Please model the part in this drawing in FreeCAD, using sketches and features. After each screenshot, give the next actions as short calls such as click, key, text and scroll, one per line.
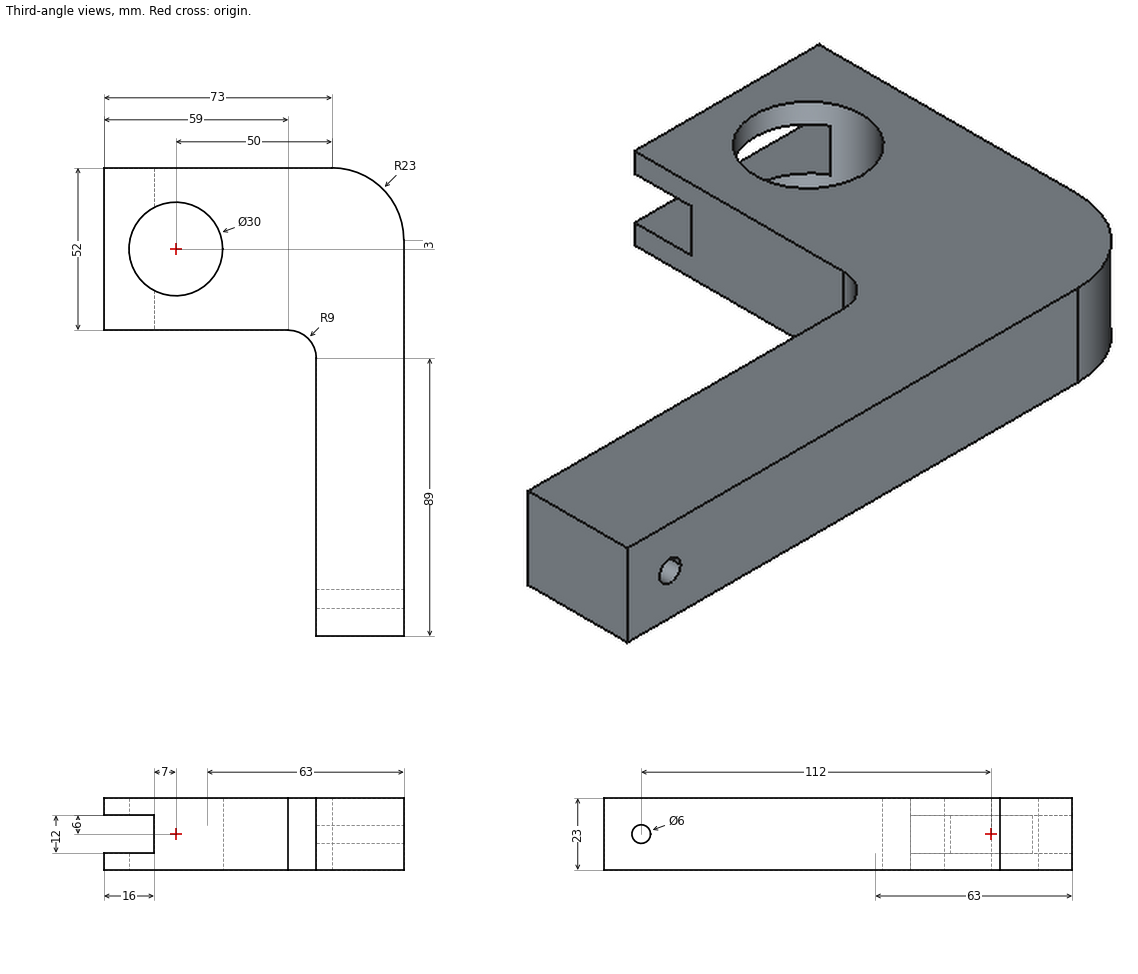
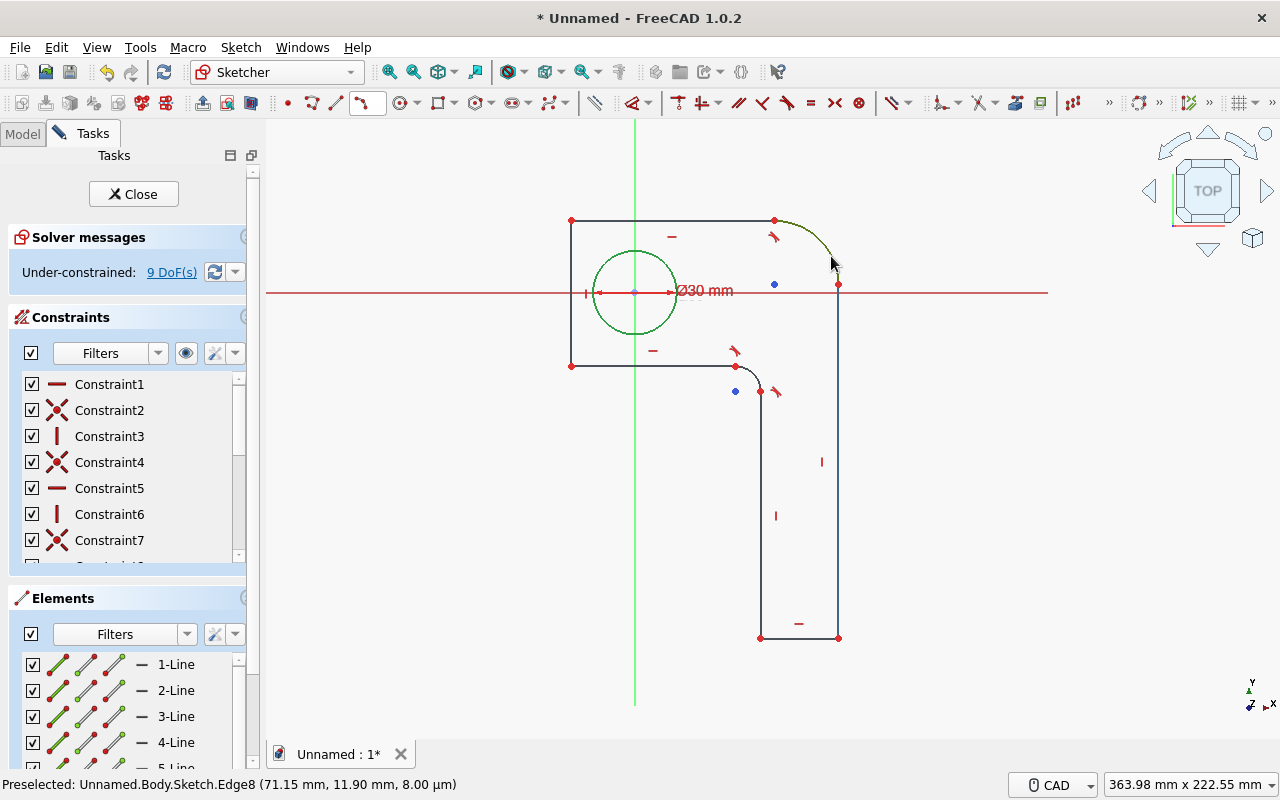
click(788, 104)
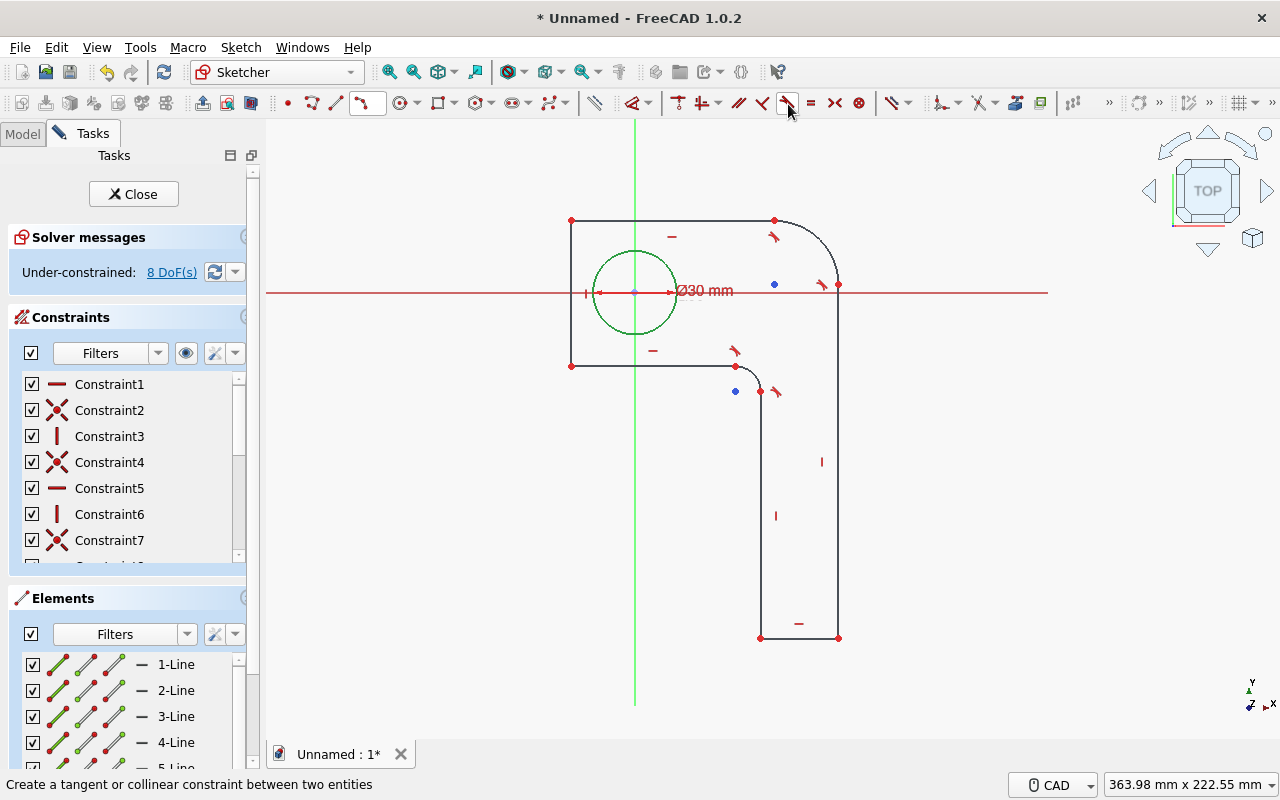
click(632, 104)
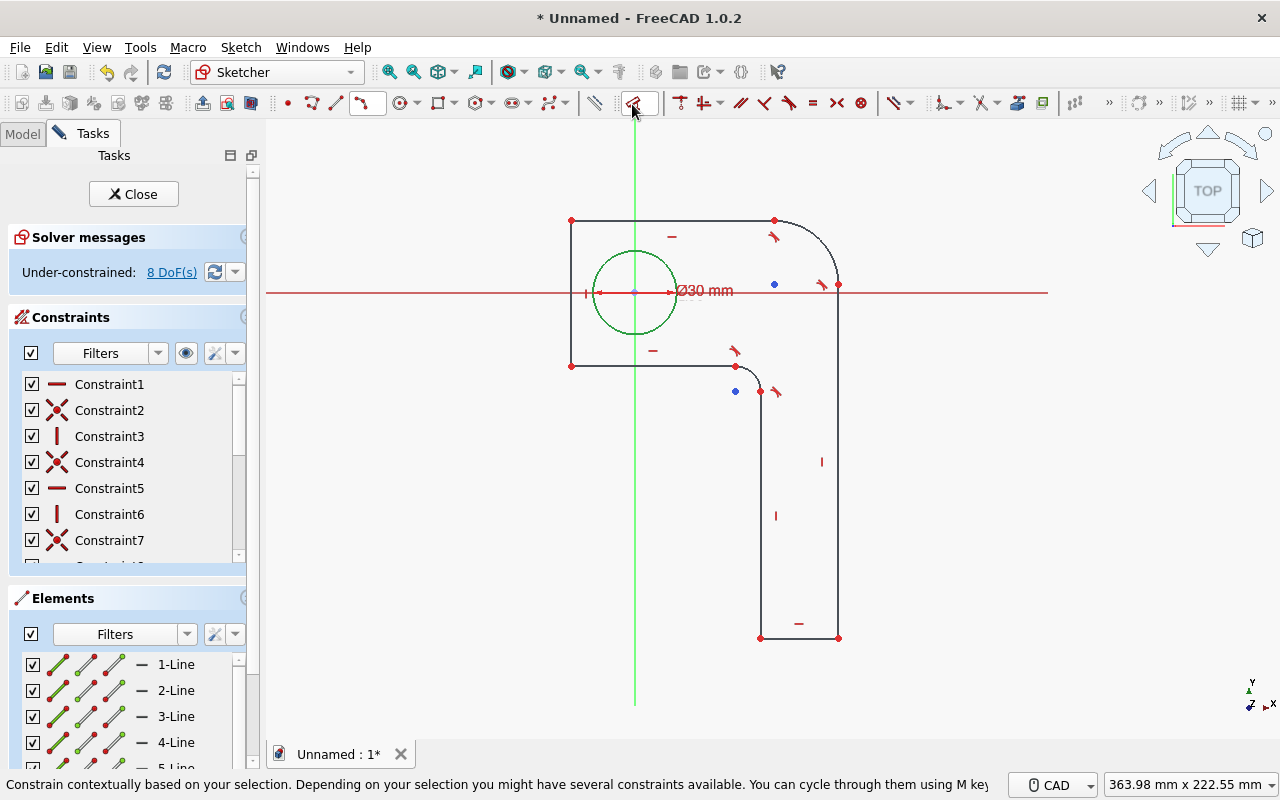
scroll(758, 380, up, 3)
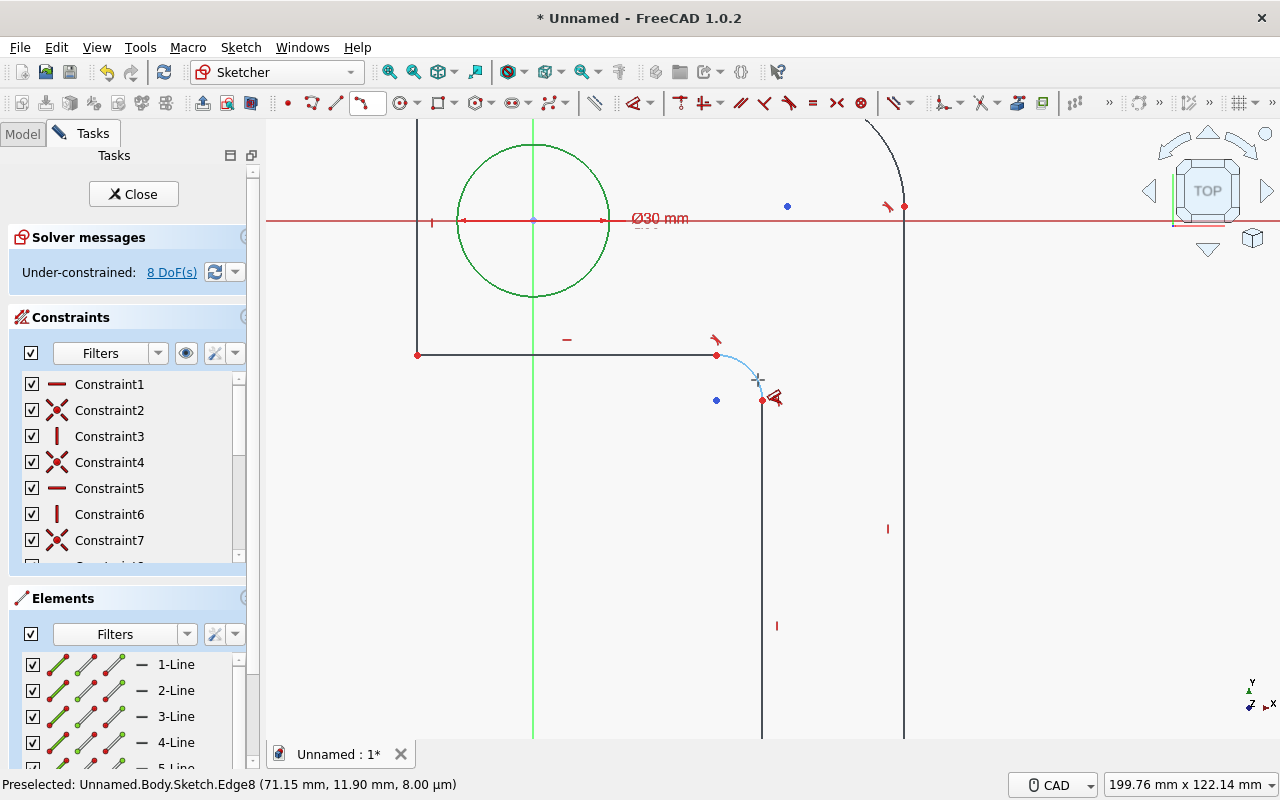
click(757, 380)
click(785, 365)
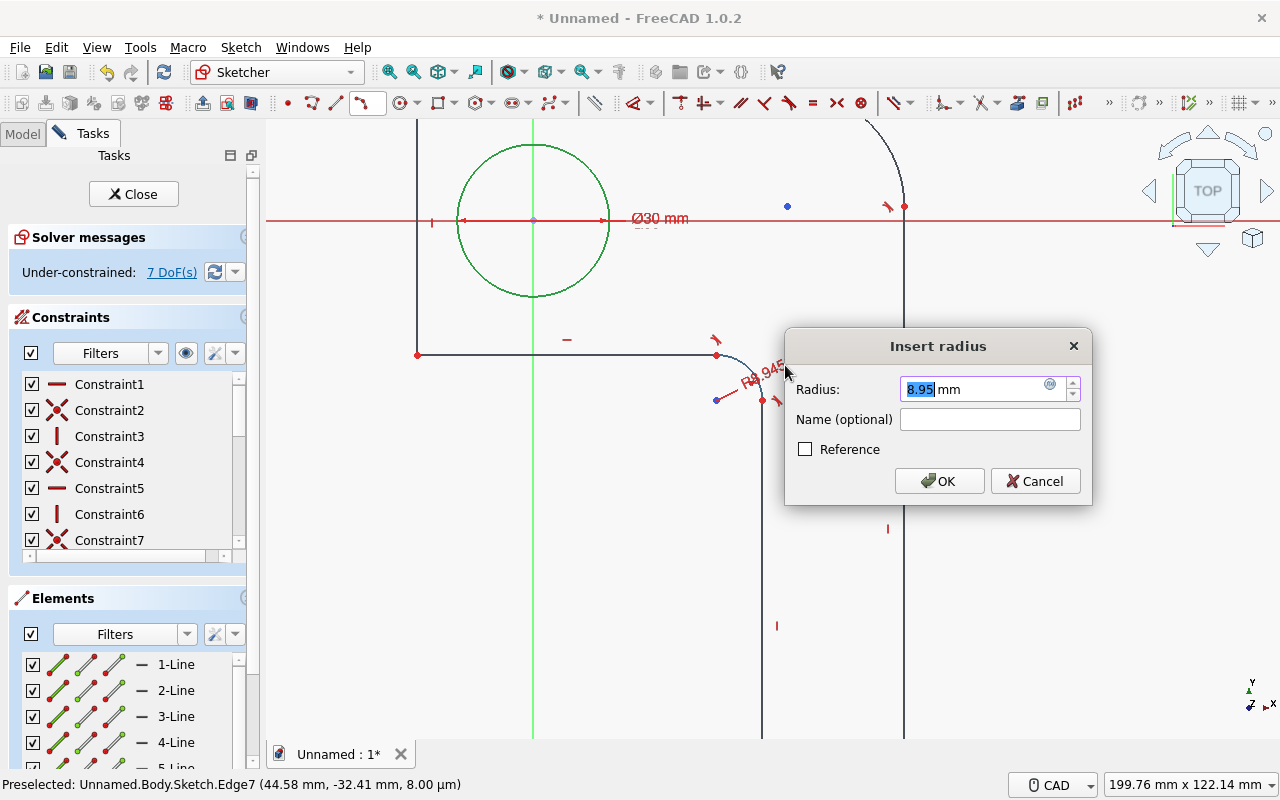
text(9)
key(Return)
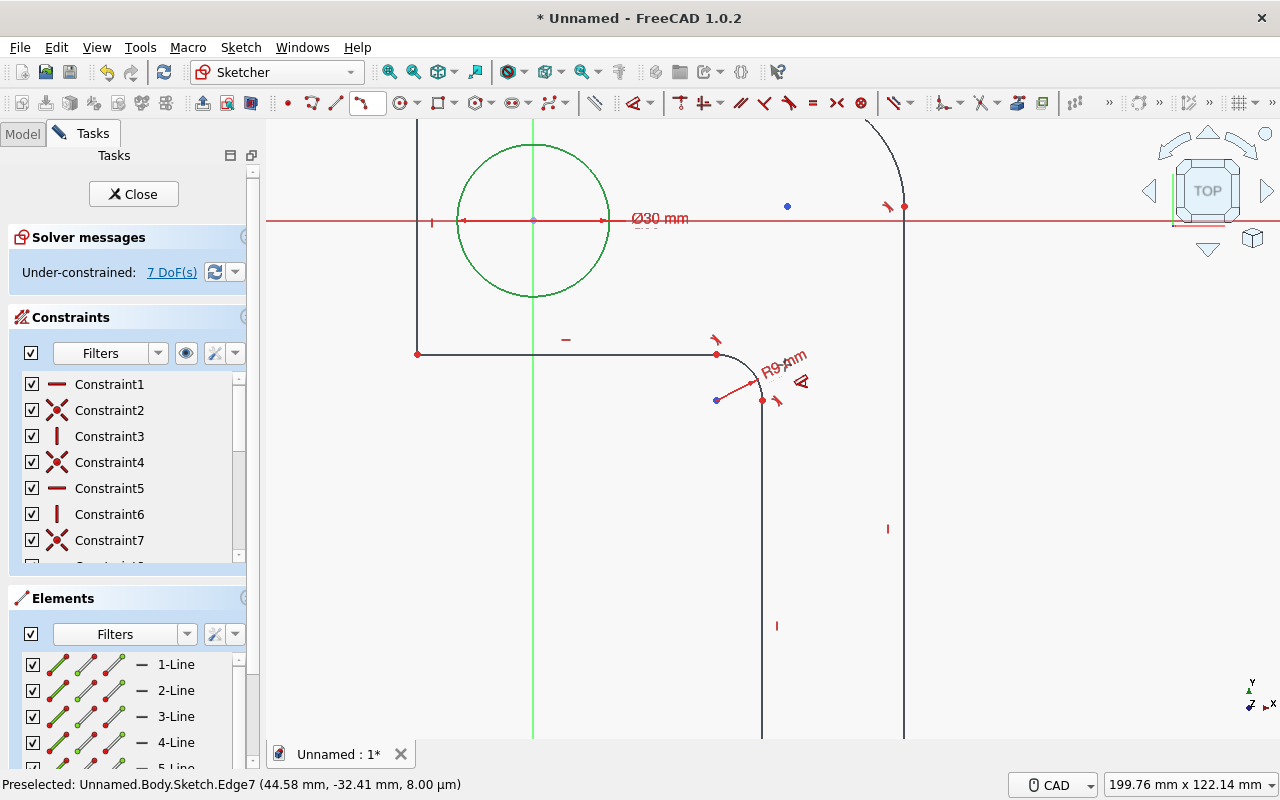
click(892, 153)
click(856, 339)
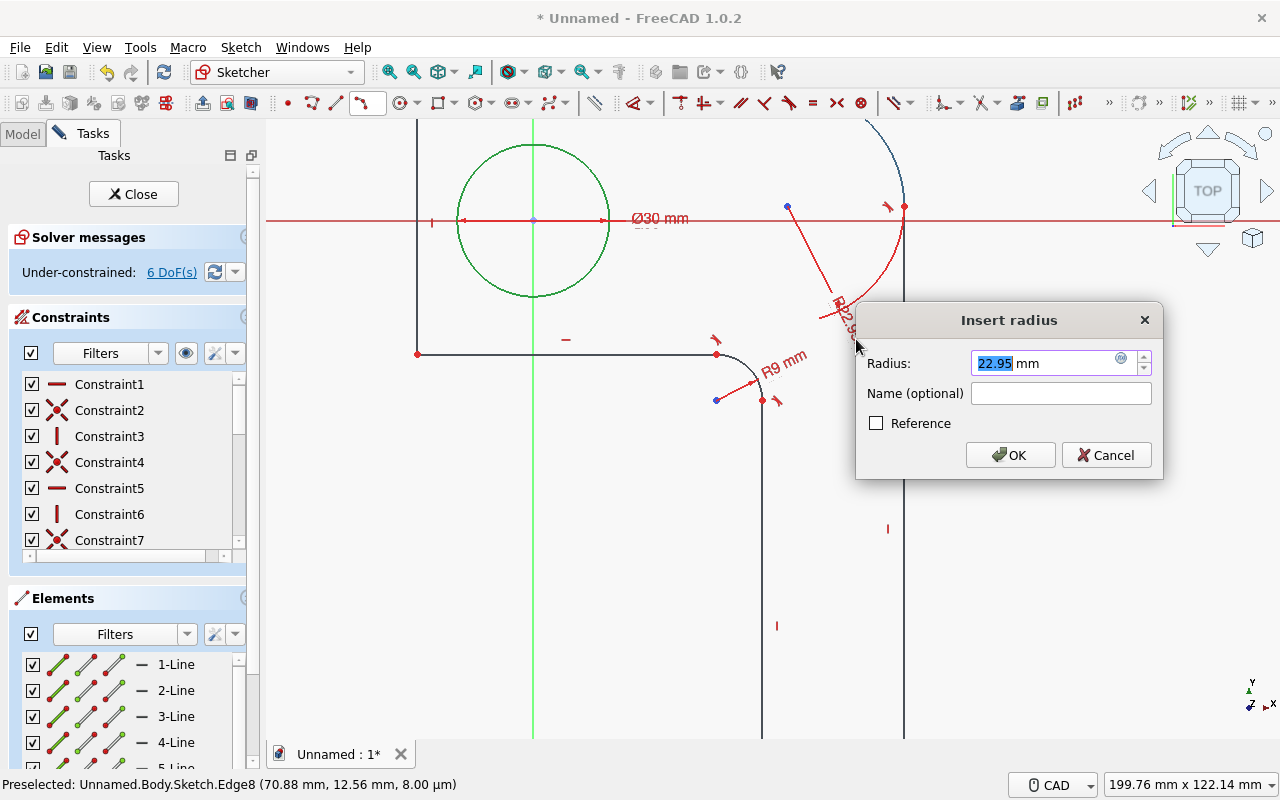
text(23)
key(Return)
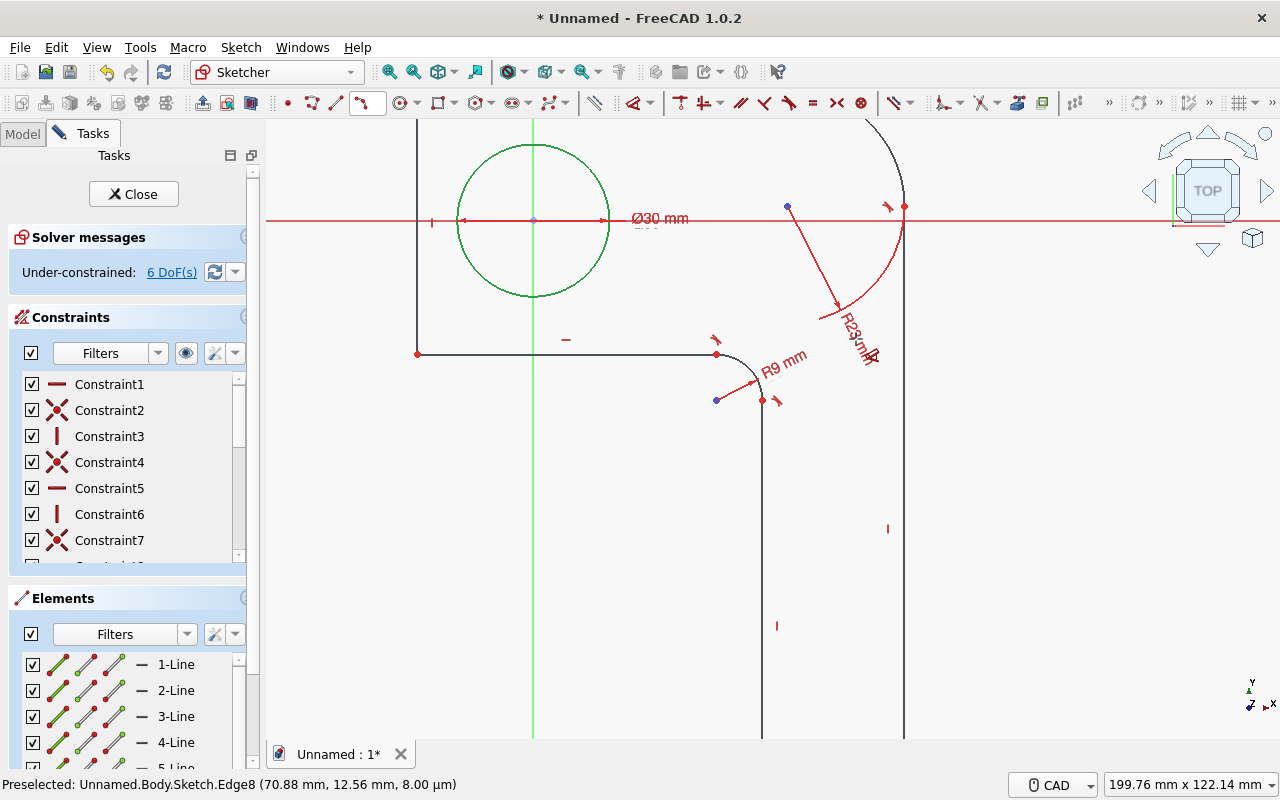
scroll(758, 380, down, 3)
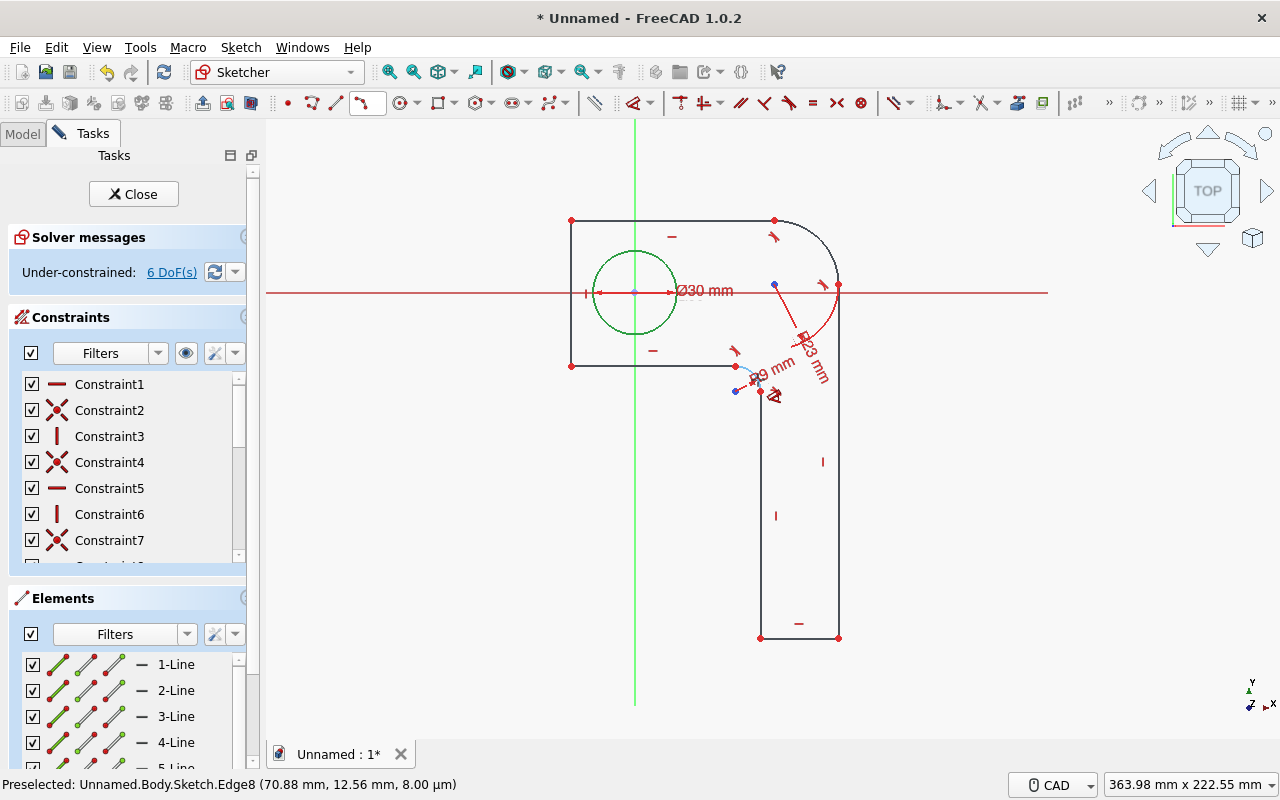
click(714, 221)
click(673, 187)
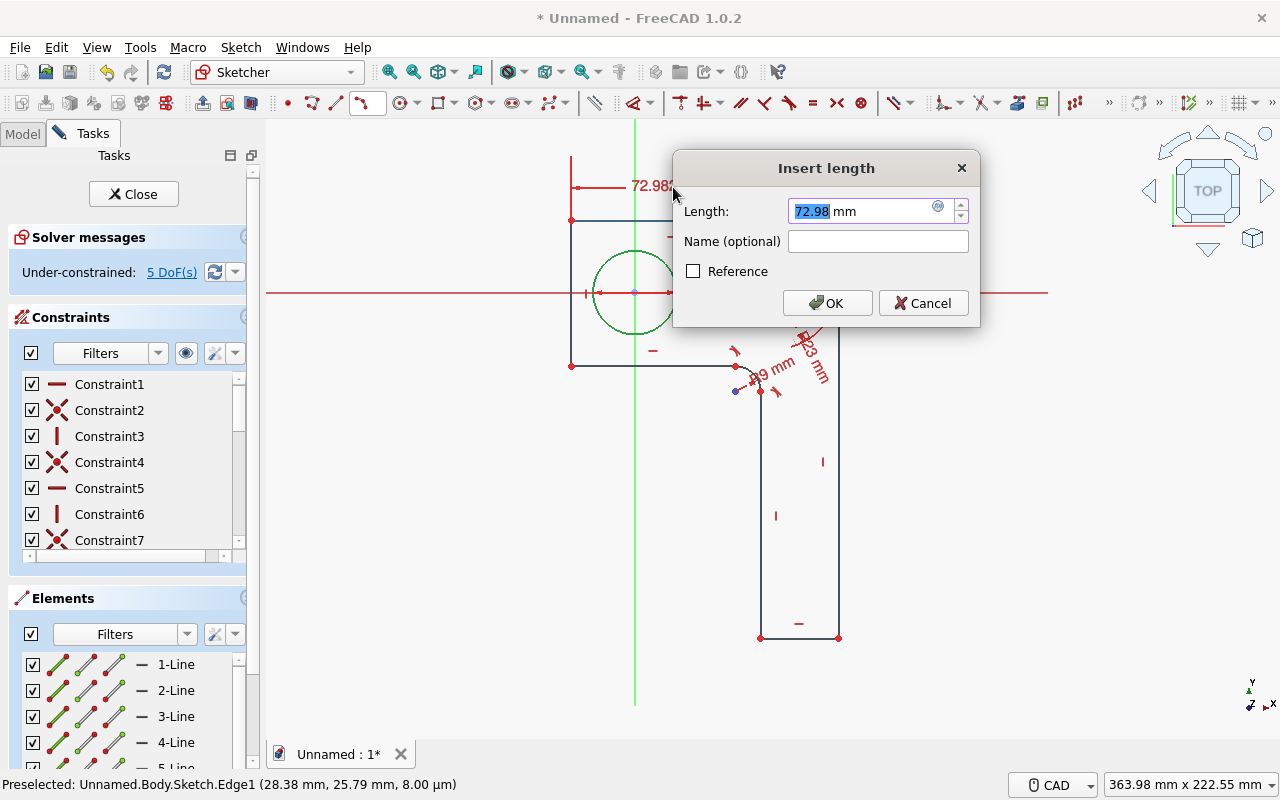
text(73)
key(Return)